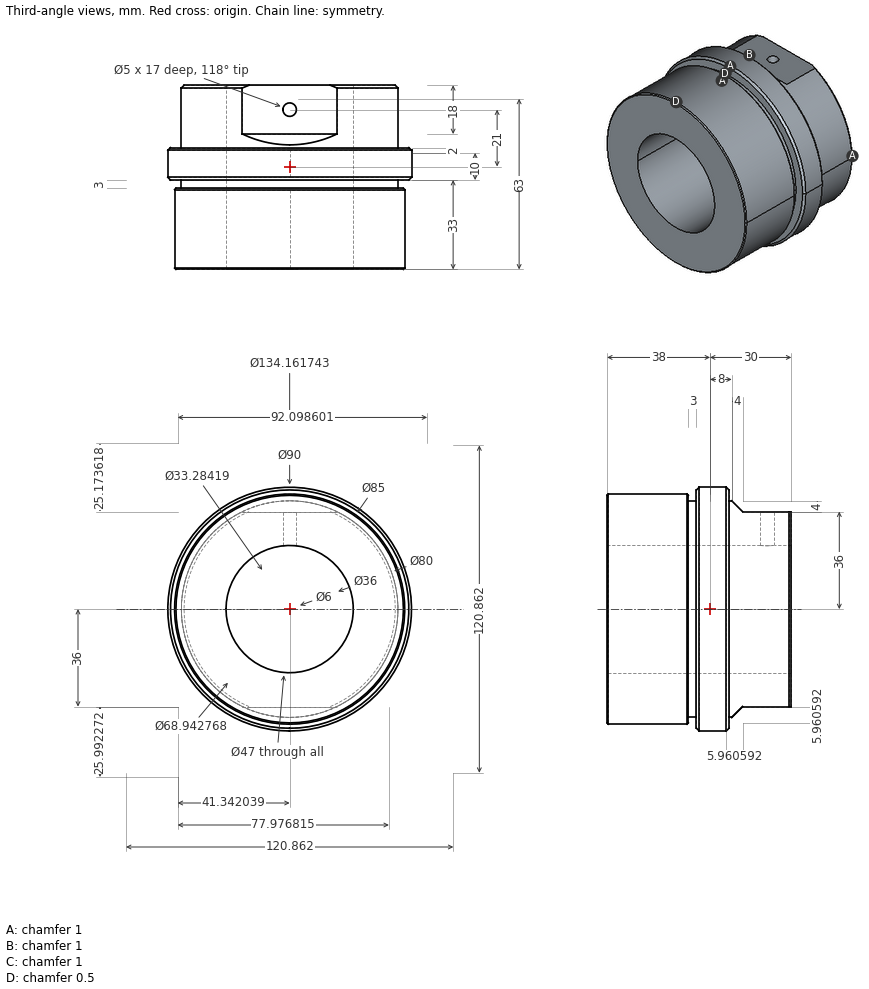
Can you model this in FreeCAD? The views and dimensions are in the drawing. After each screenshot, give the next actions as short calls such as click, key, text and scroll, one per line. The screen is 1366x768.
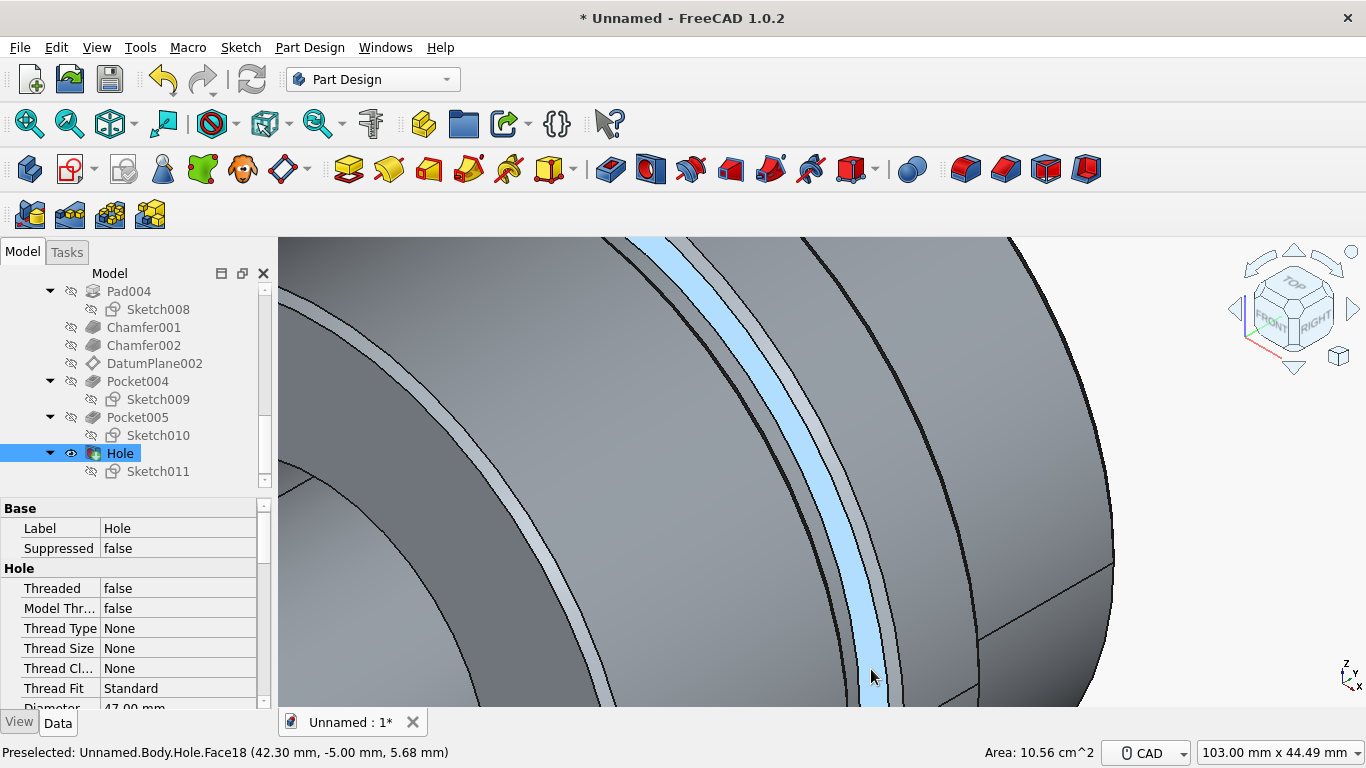
click(70, 170)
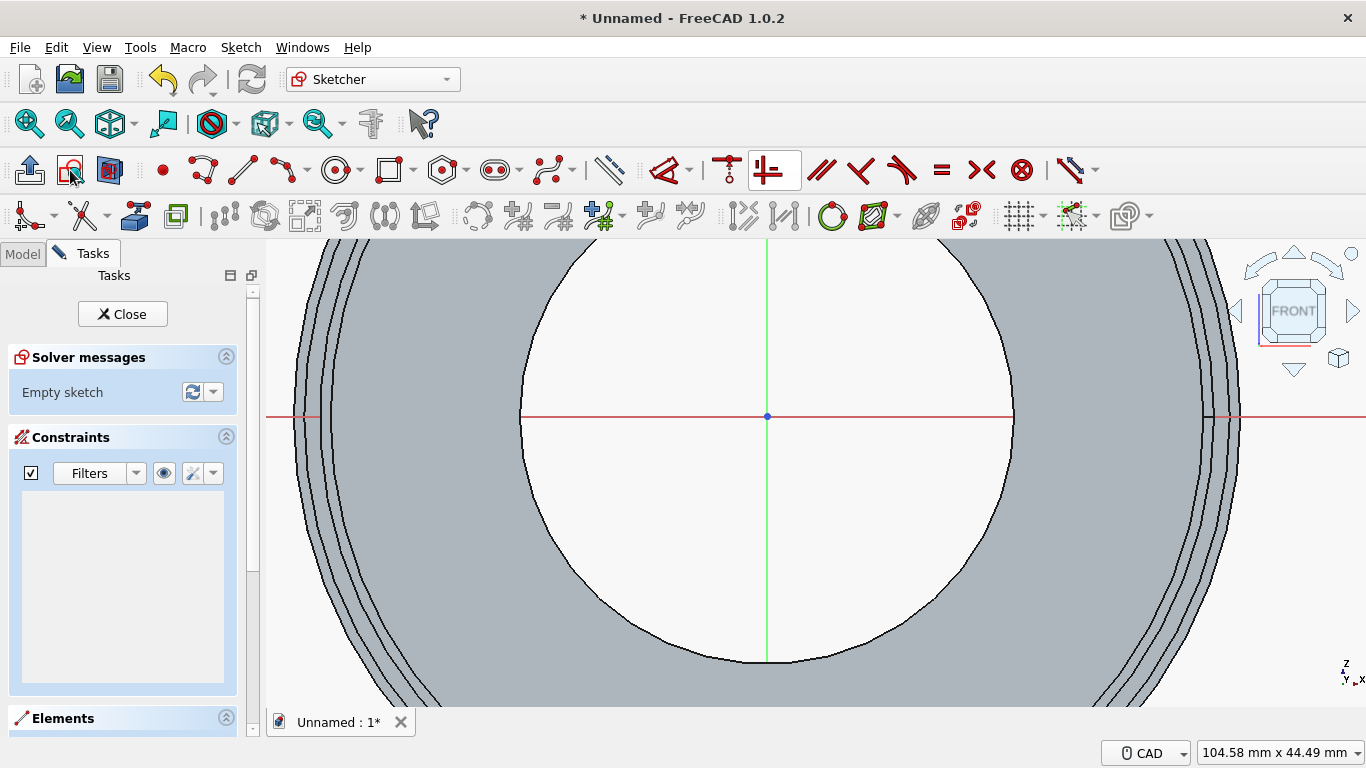
scroll(739, 497, down, 6)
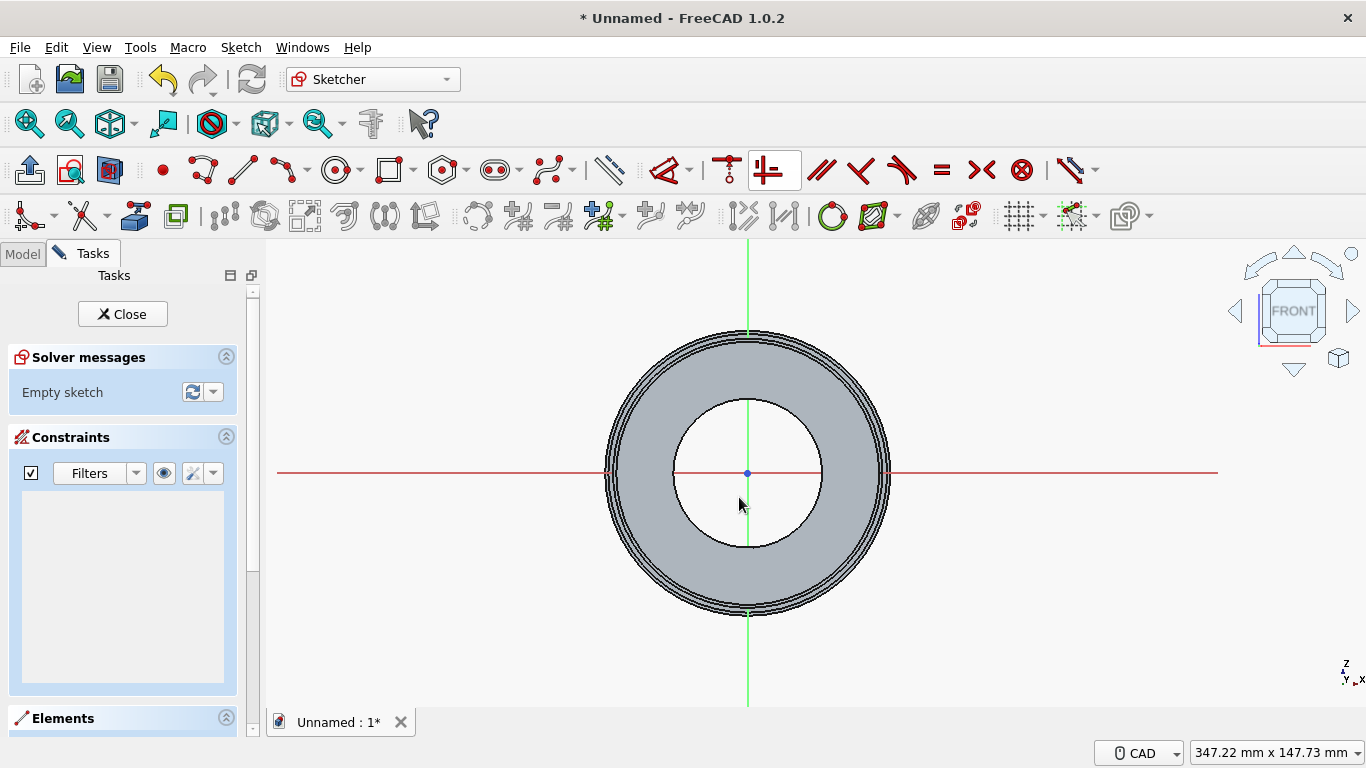
click(336, 170)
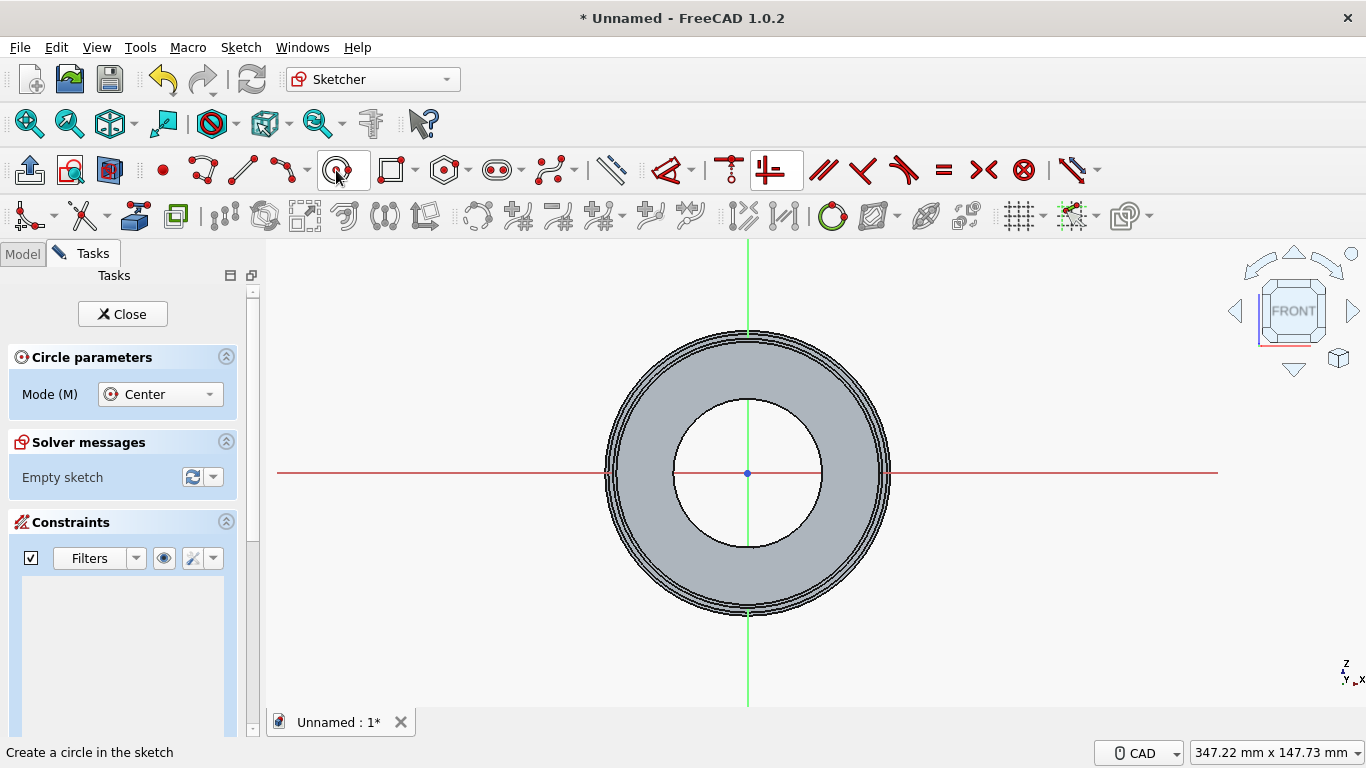
click(748, 473)
click(843, 378)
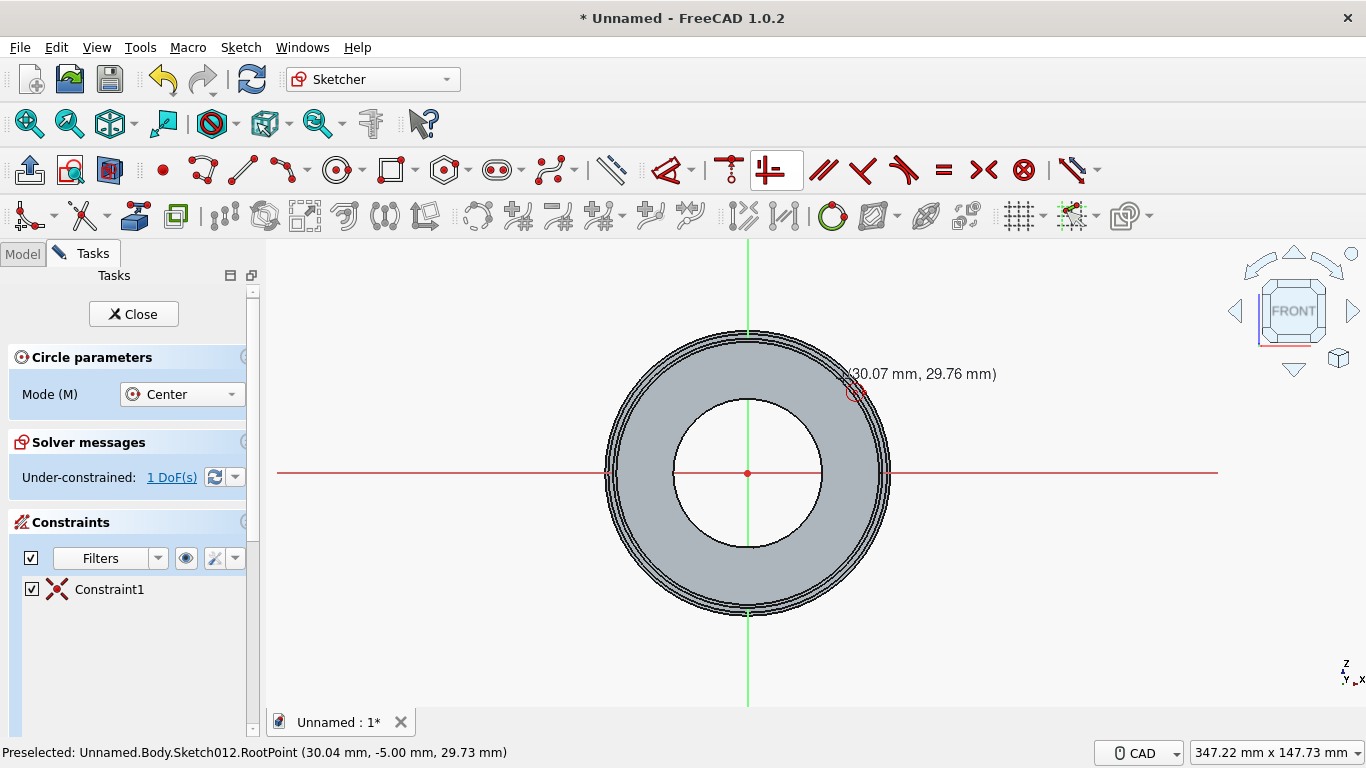
click(748, 473)
click(825, 396)
key(Escape)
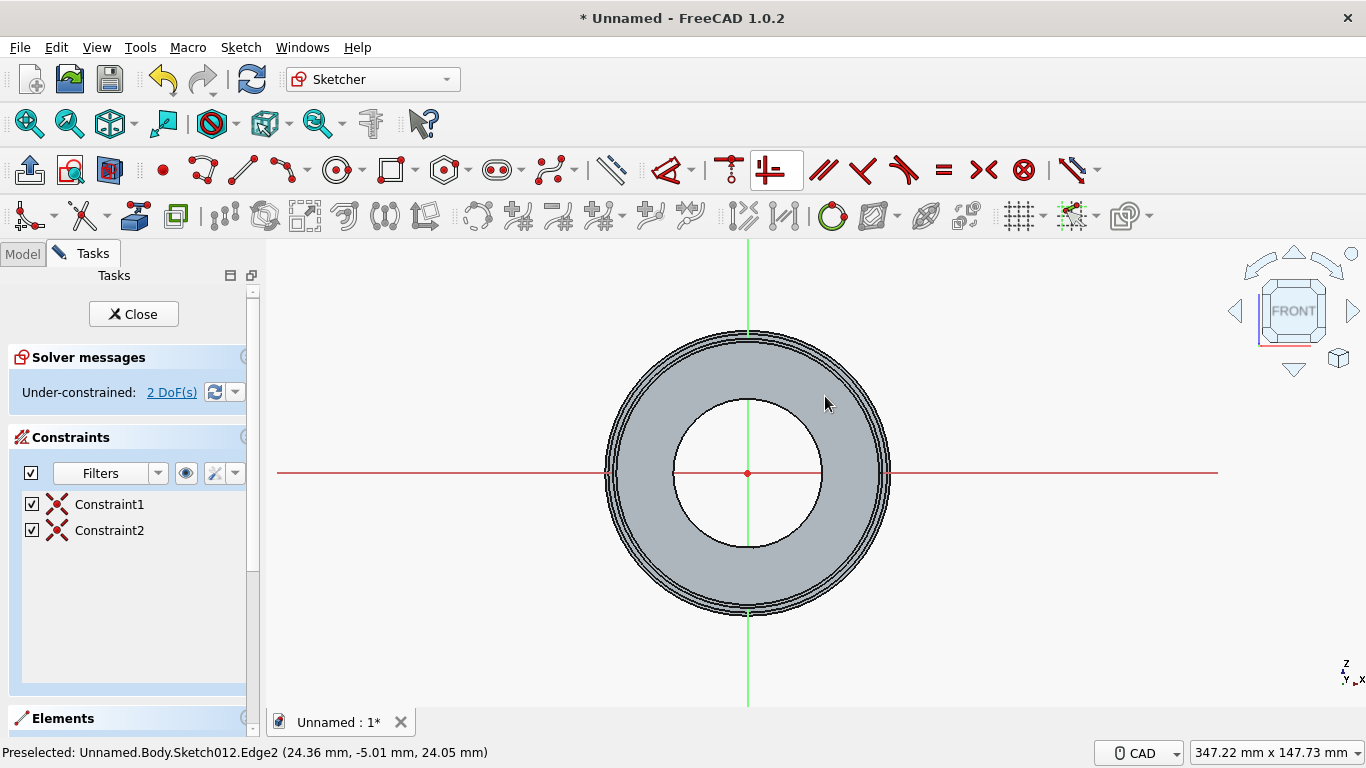
click(666, 170)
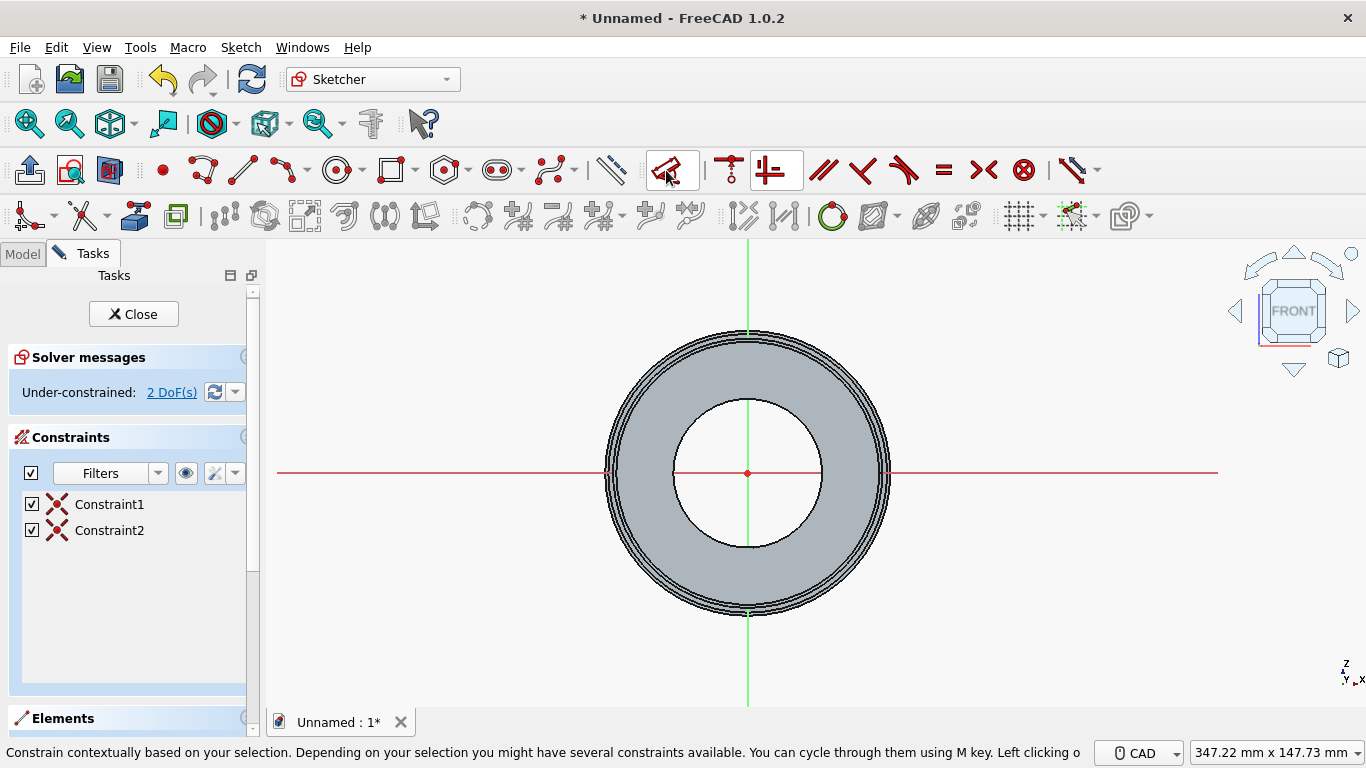
click(842, 378)
click(865, 355)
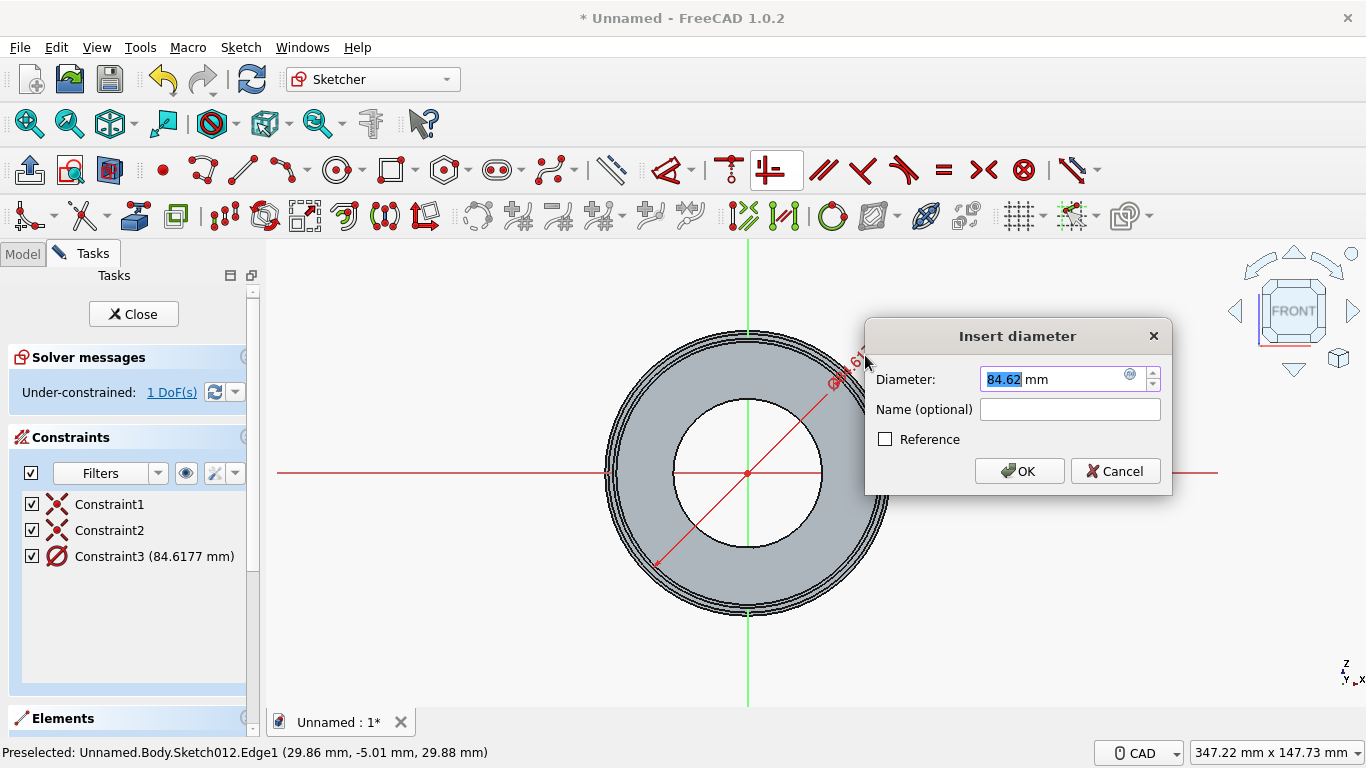
text(85)
key(Return)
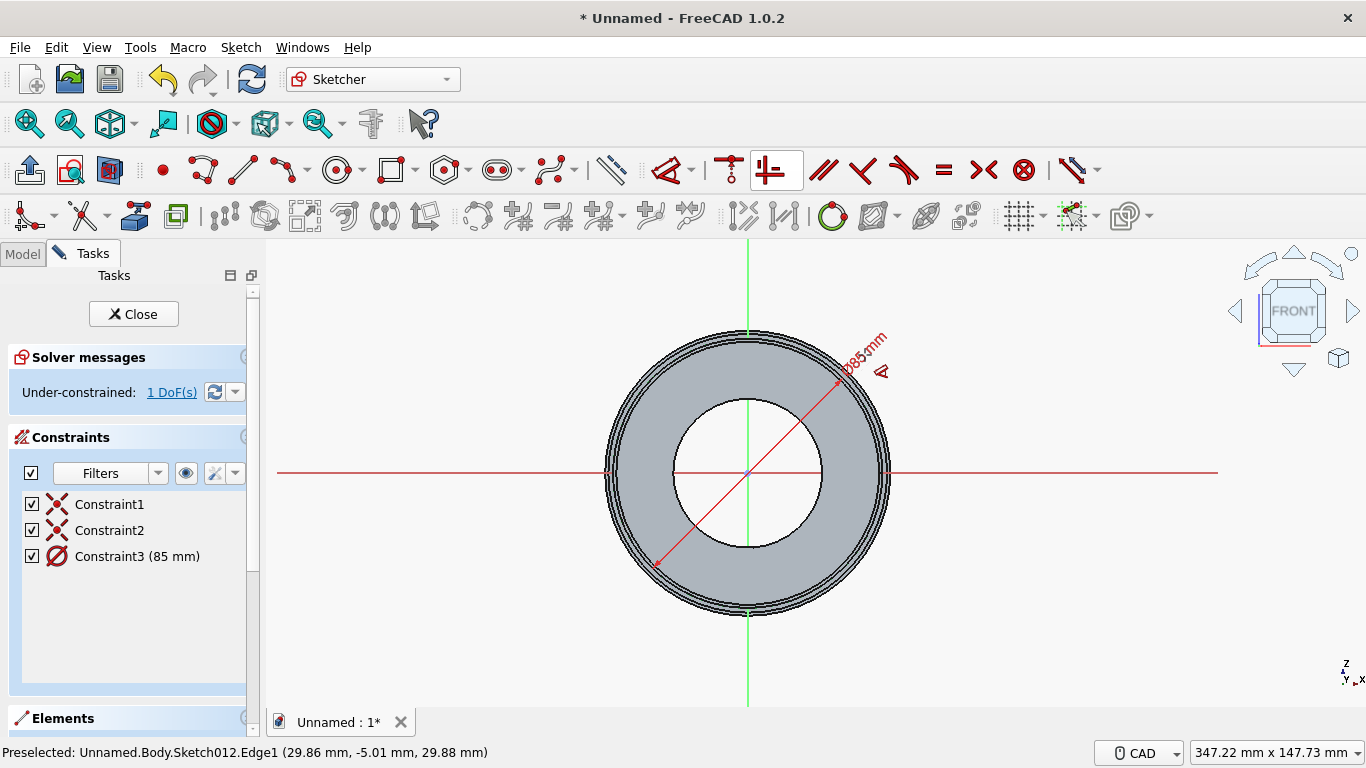
click(824, 396)
click(904, 426)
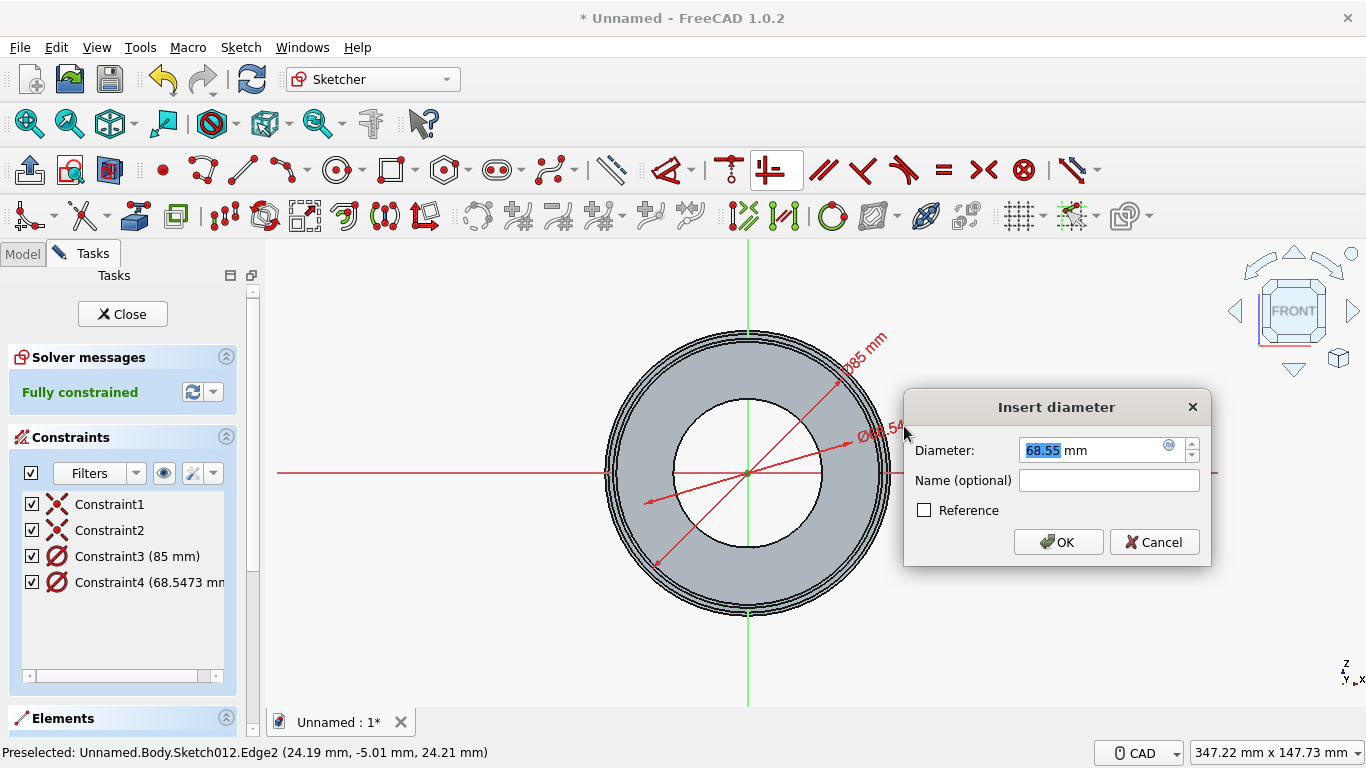
text(68.942768)
key(Return)
key(Escape)